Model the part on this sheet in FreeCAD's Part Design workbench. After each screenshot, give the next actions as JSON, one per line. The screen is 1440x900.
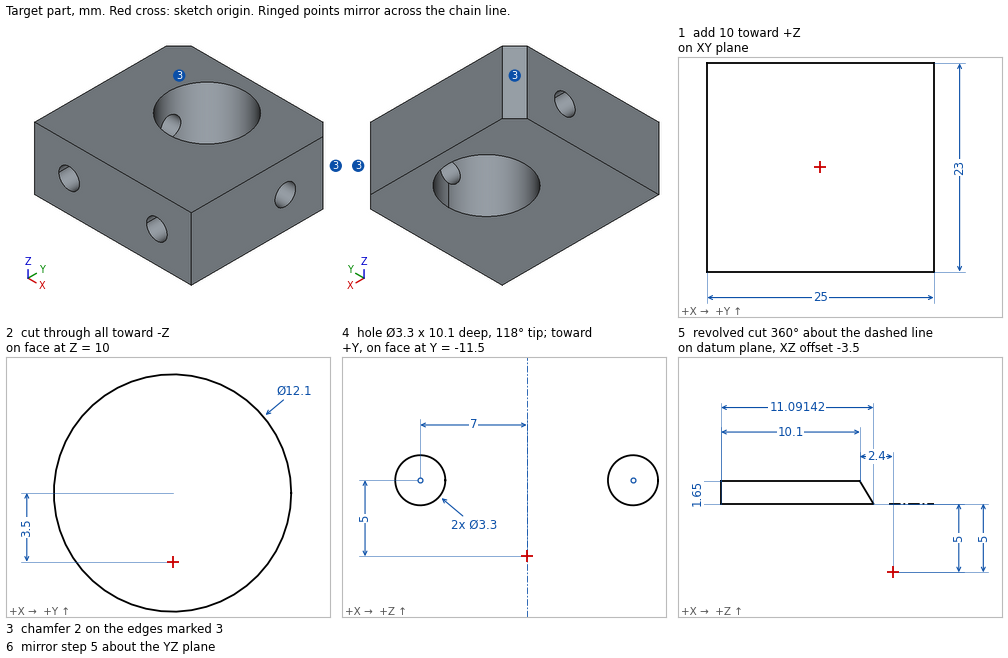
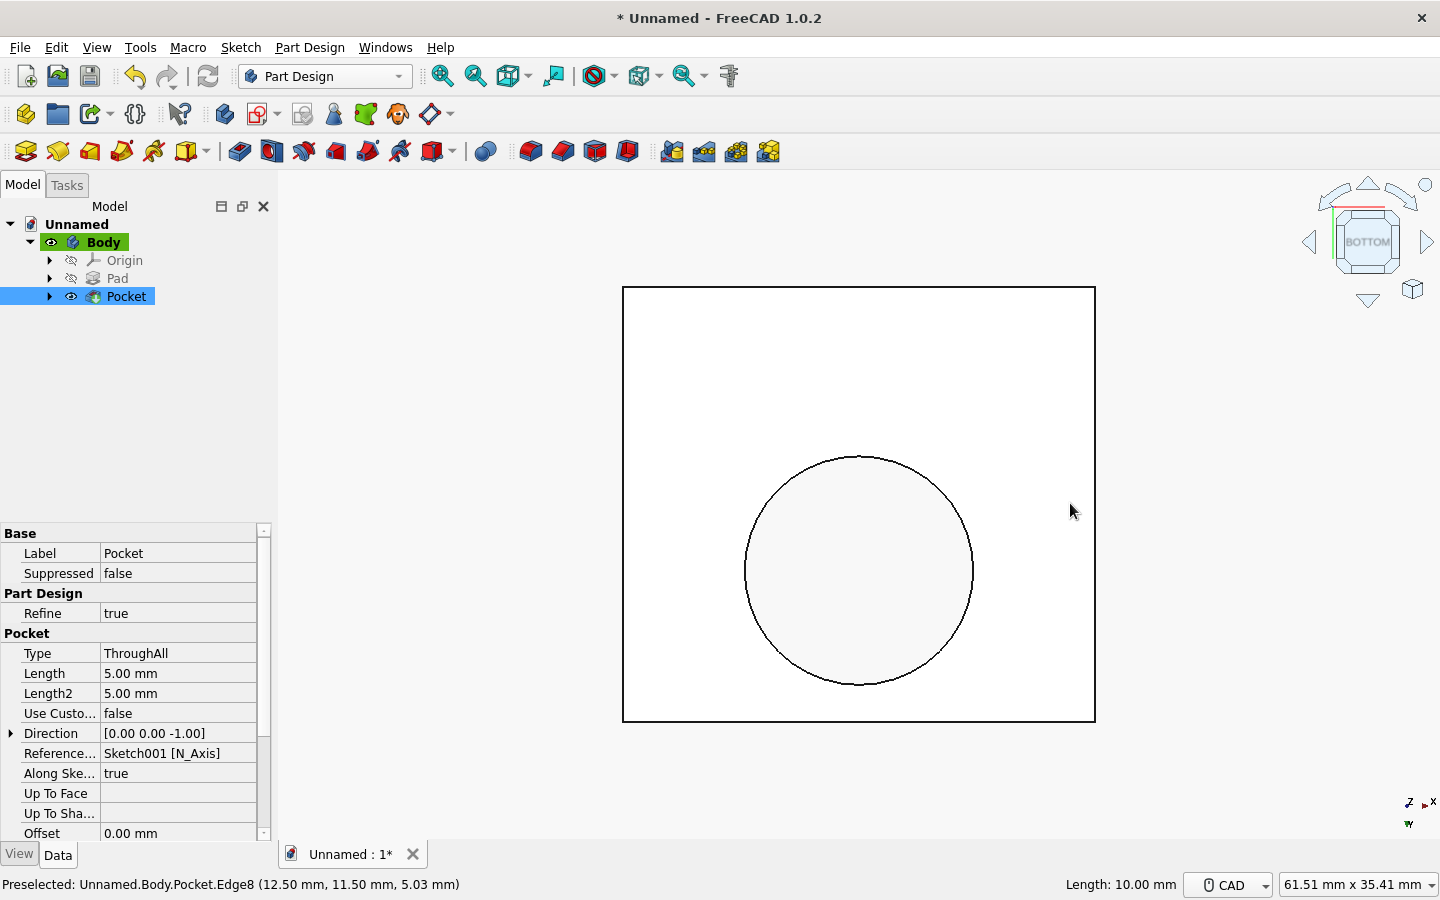
{"action": "key", "text": "4"}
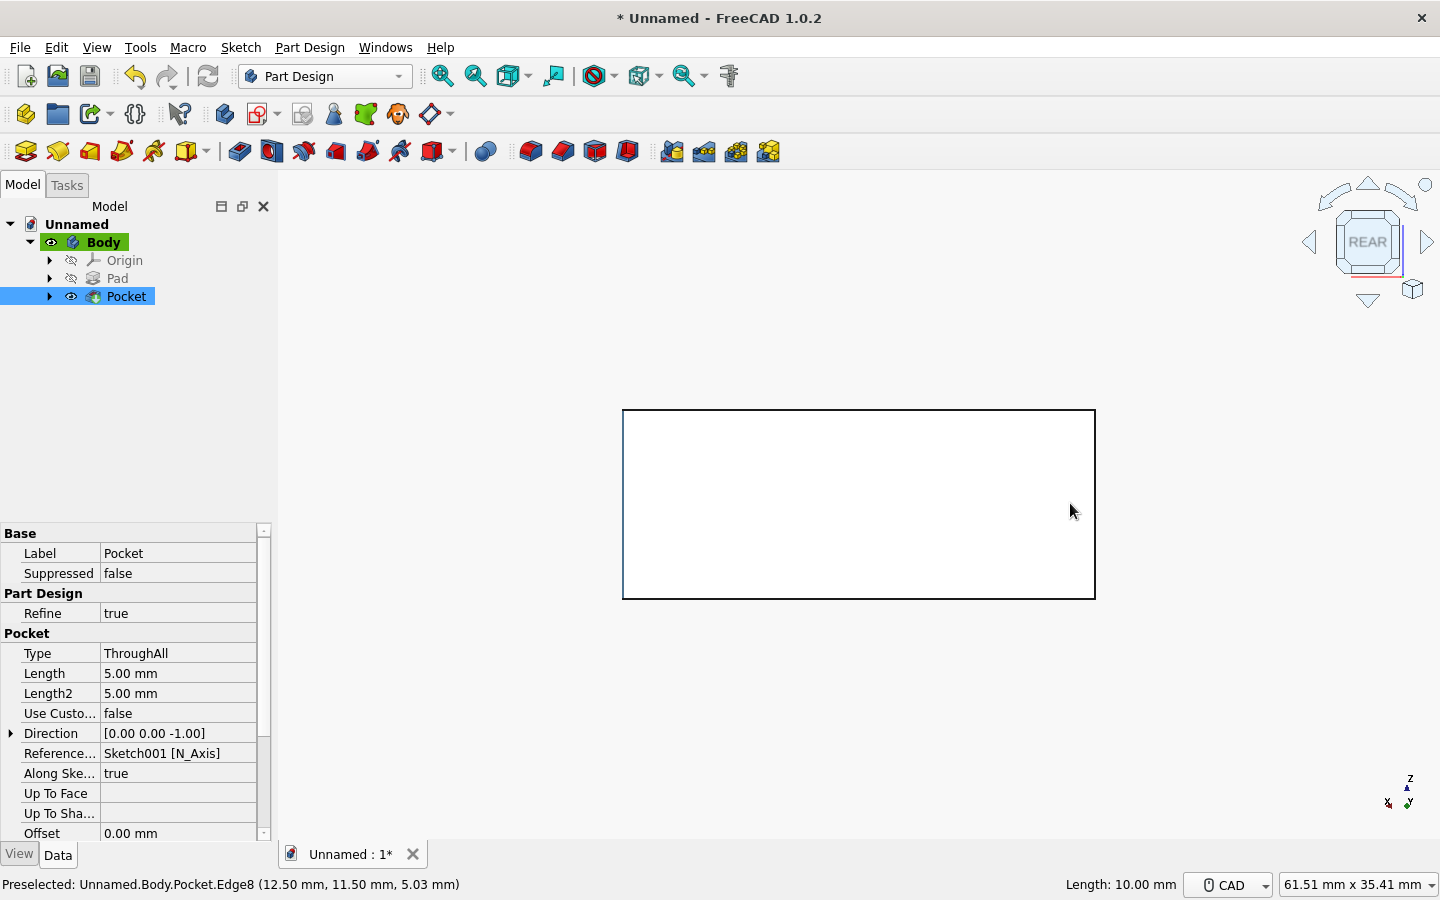
{"action": "left_click", "coordinate": [444, 76]}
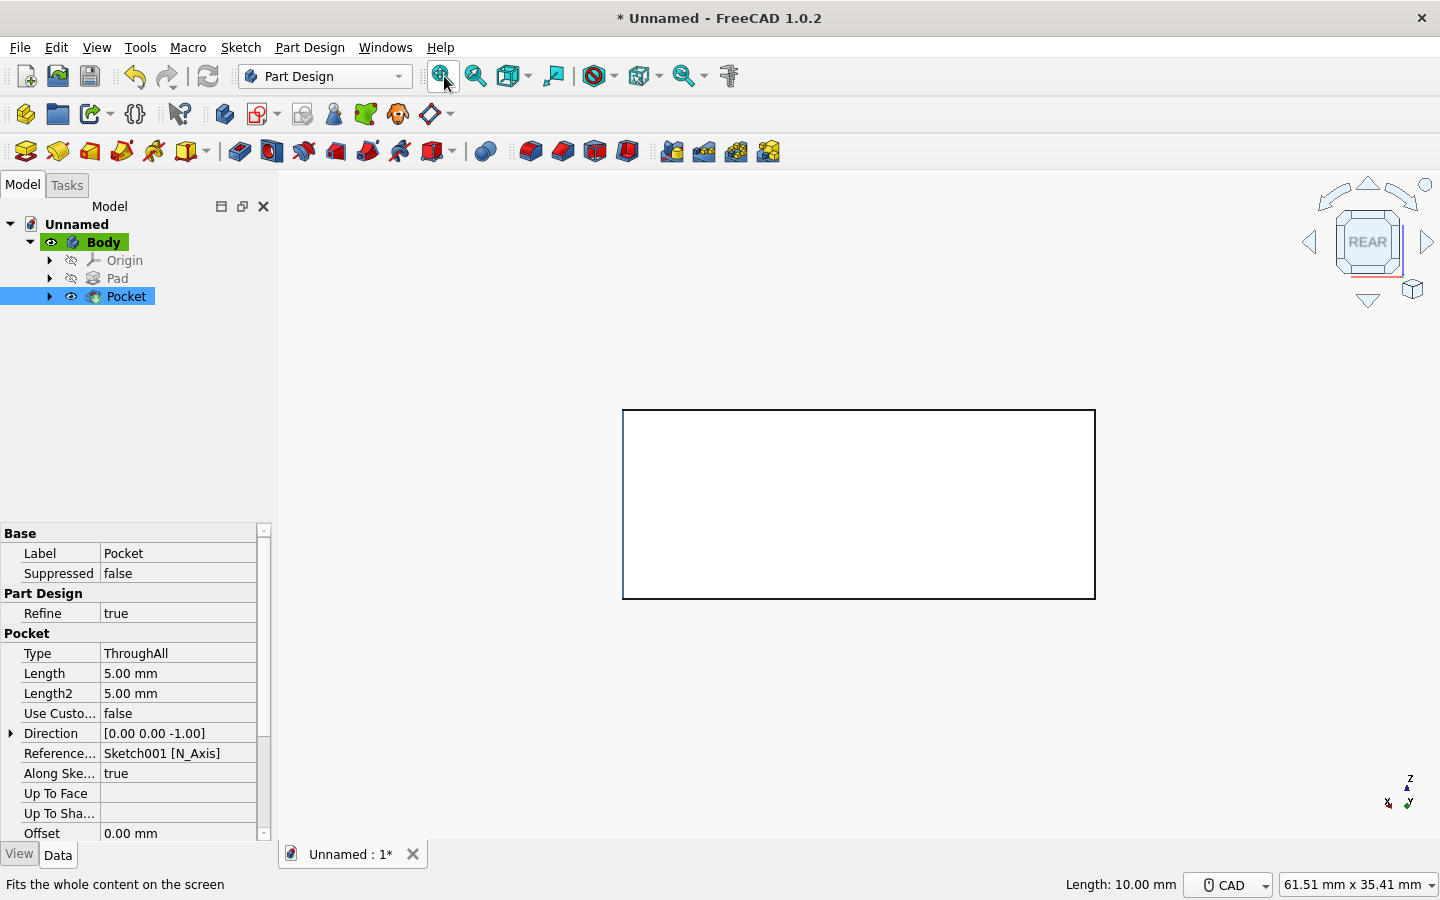
{"action": "left_click", "coordinate": [1095, 504], "text": "ctrl"}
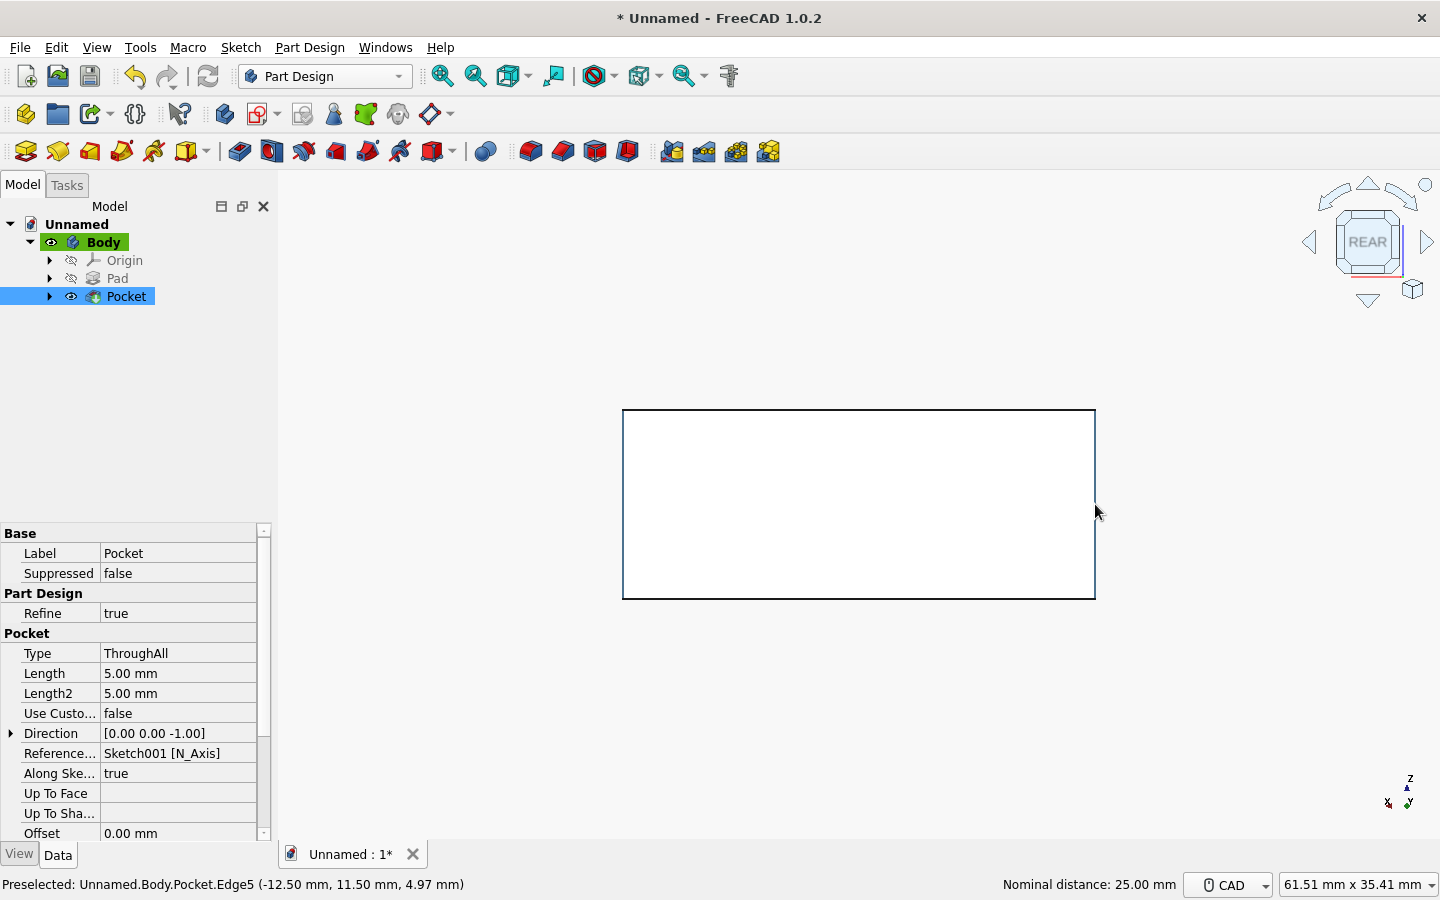
{"action": "left_click", "coordinate": [564, 152]}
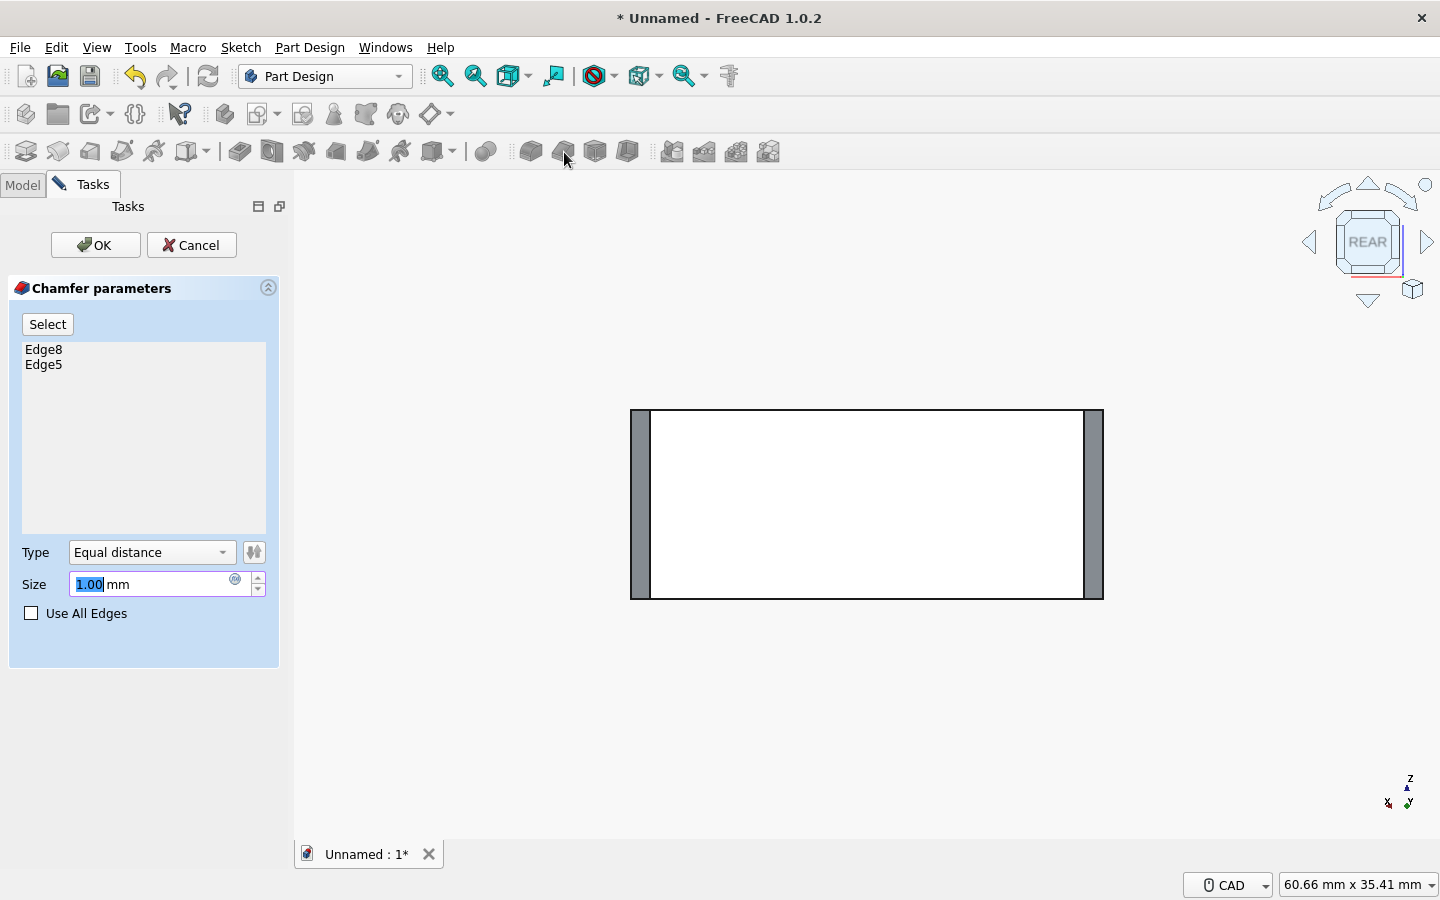
{"action": "type", "text": "2"}
{"action": "key", "text": "Tab"}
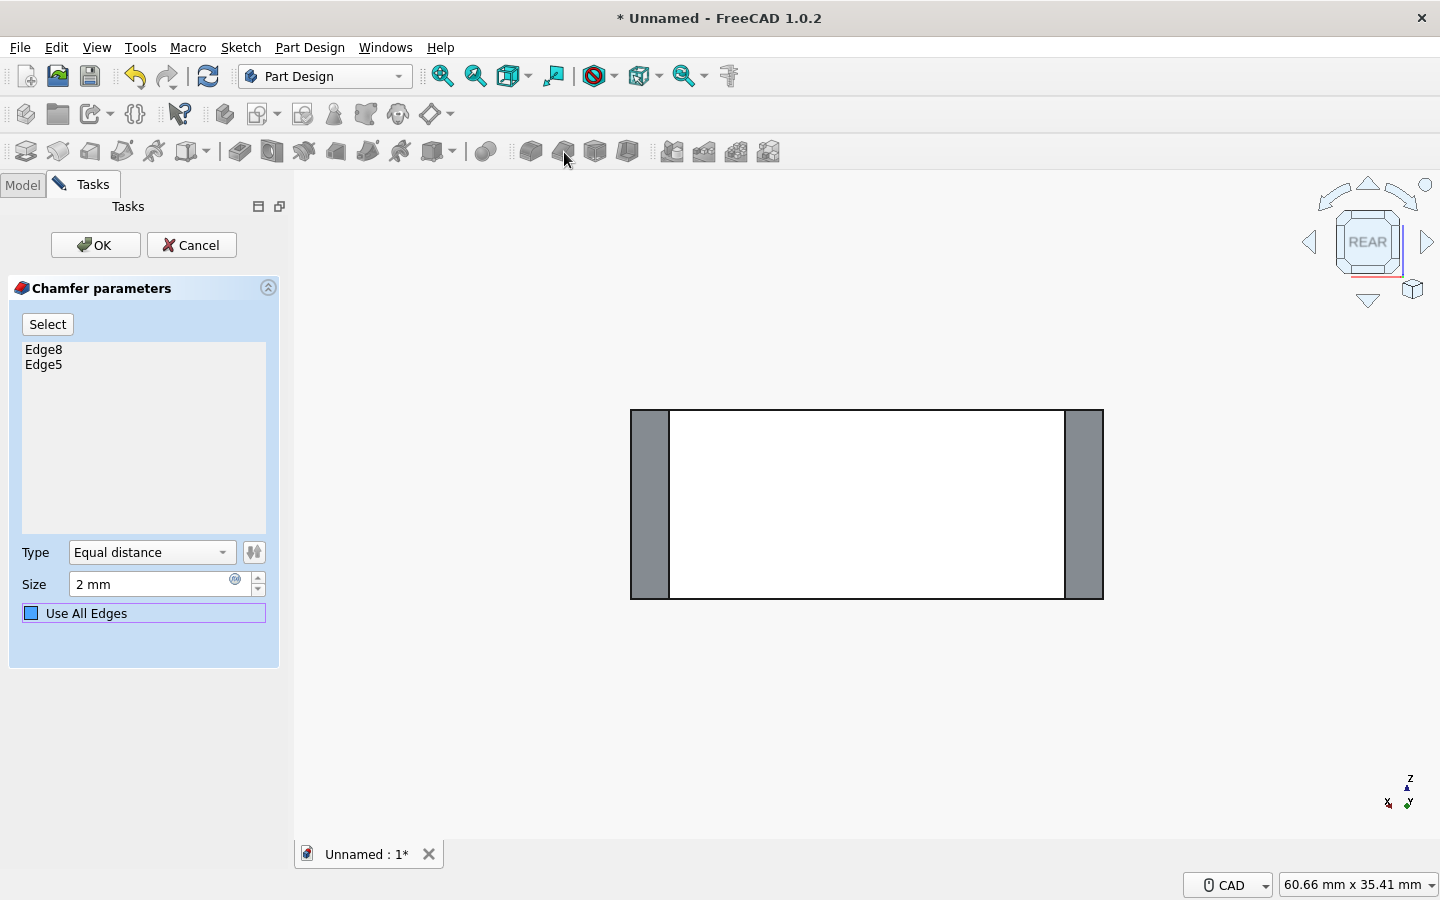
{"action": "left_click", "coordinate": [96, 245]}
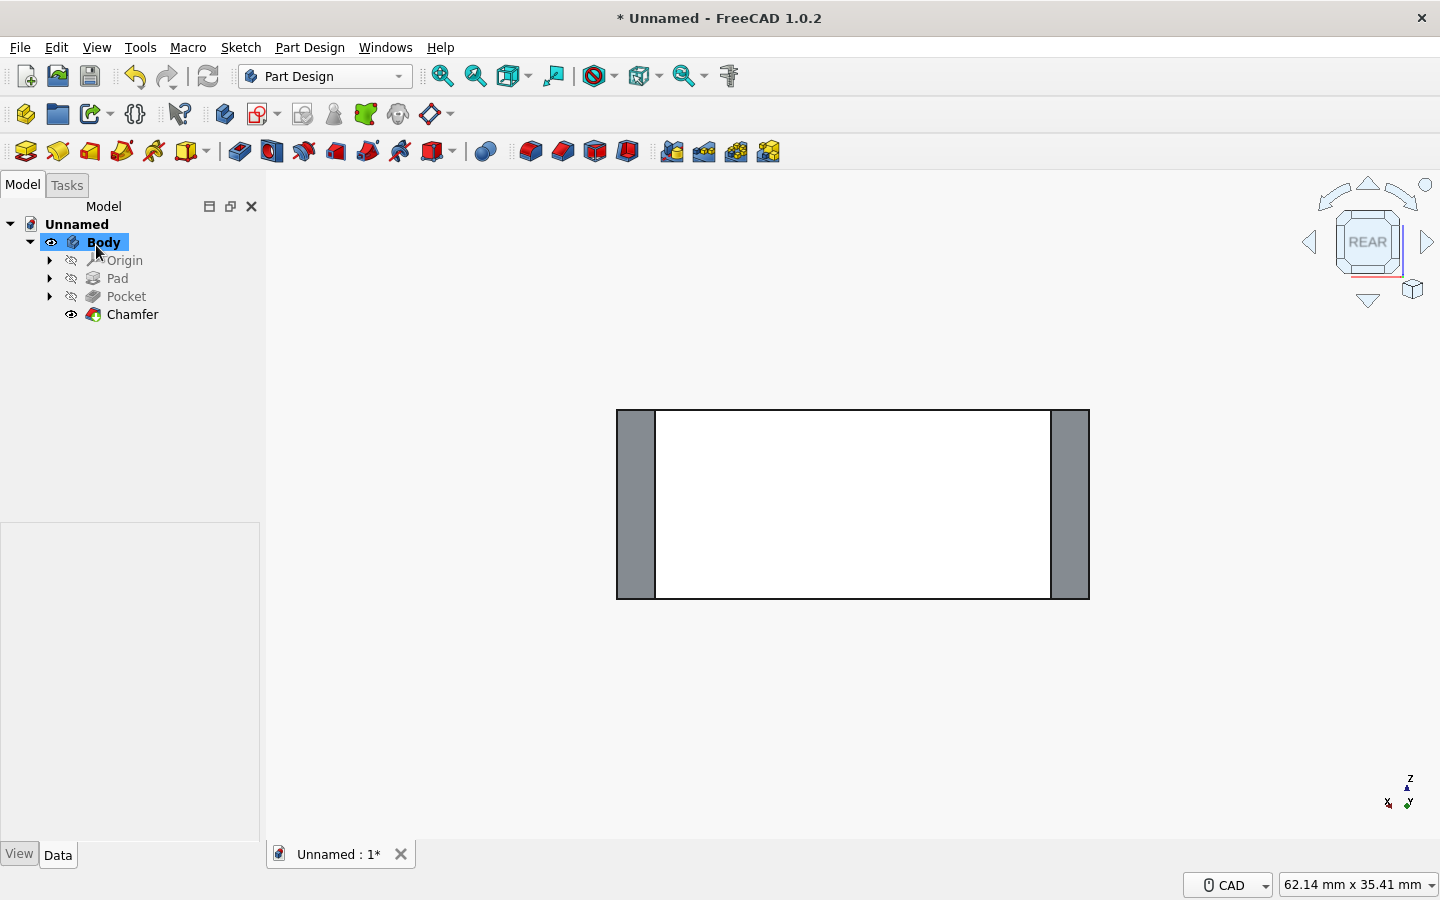
{"action": "key", "text": "v f"}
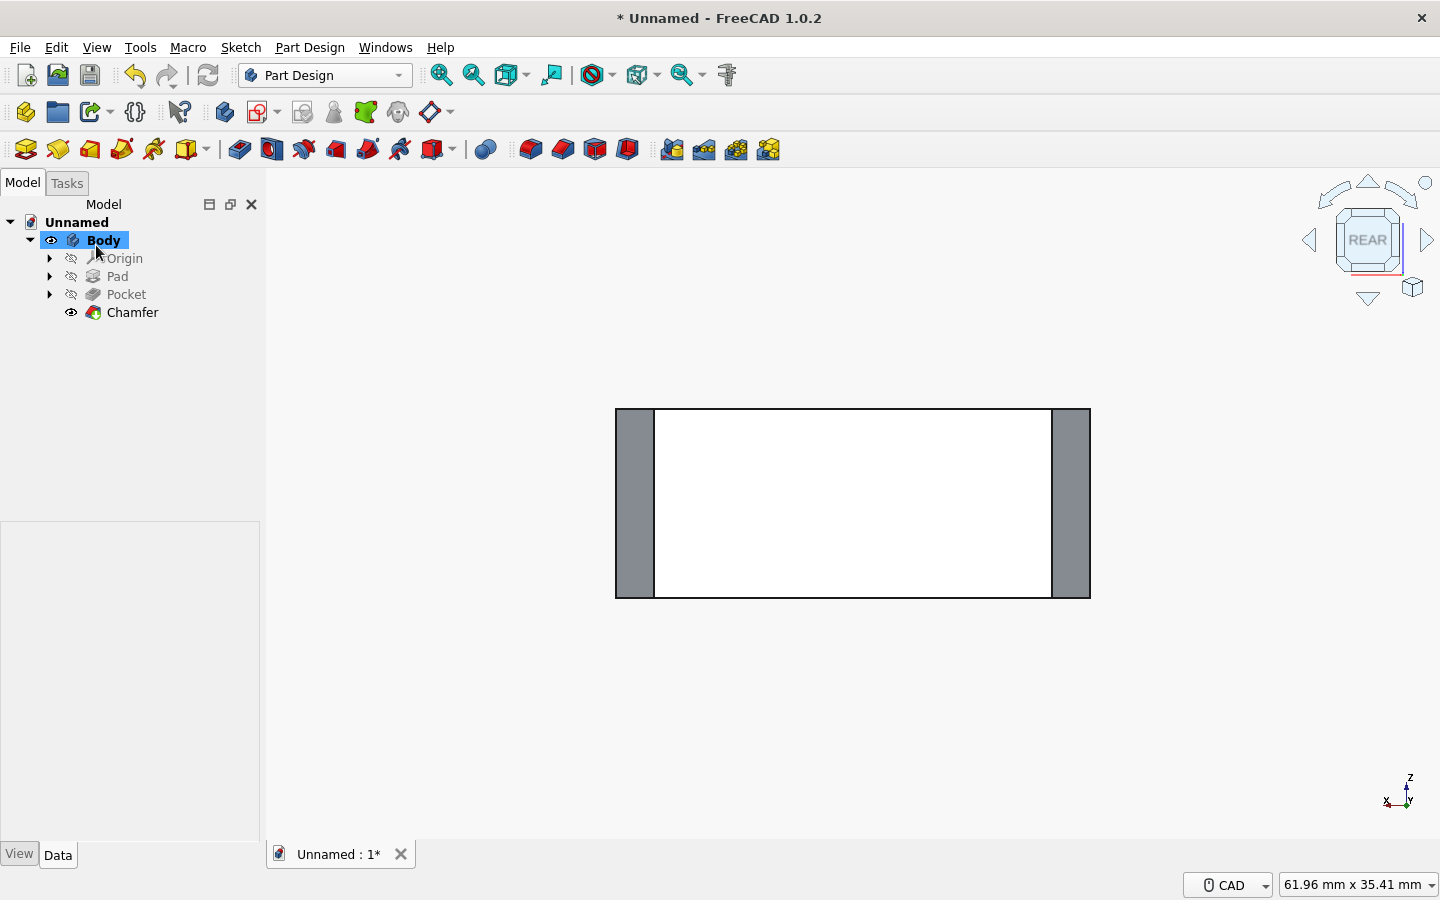
{"action": "key", "text": "0"}